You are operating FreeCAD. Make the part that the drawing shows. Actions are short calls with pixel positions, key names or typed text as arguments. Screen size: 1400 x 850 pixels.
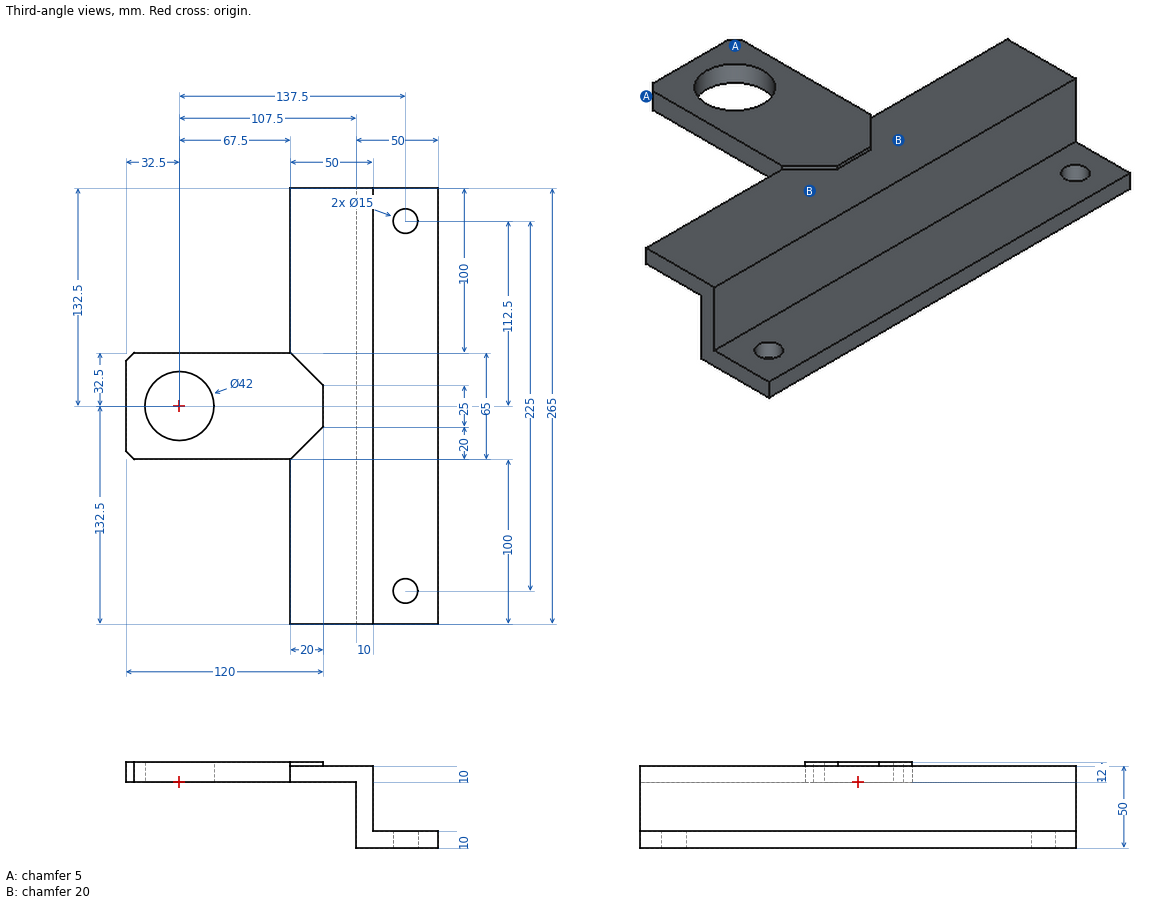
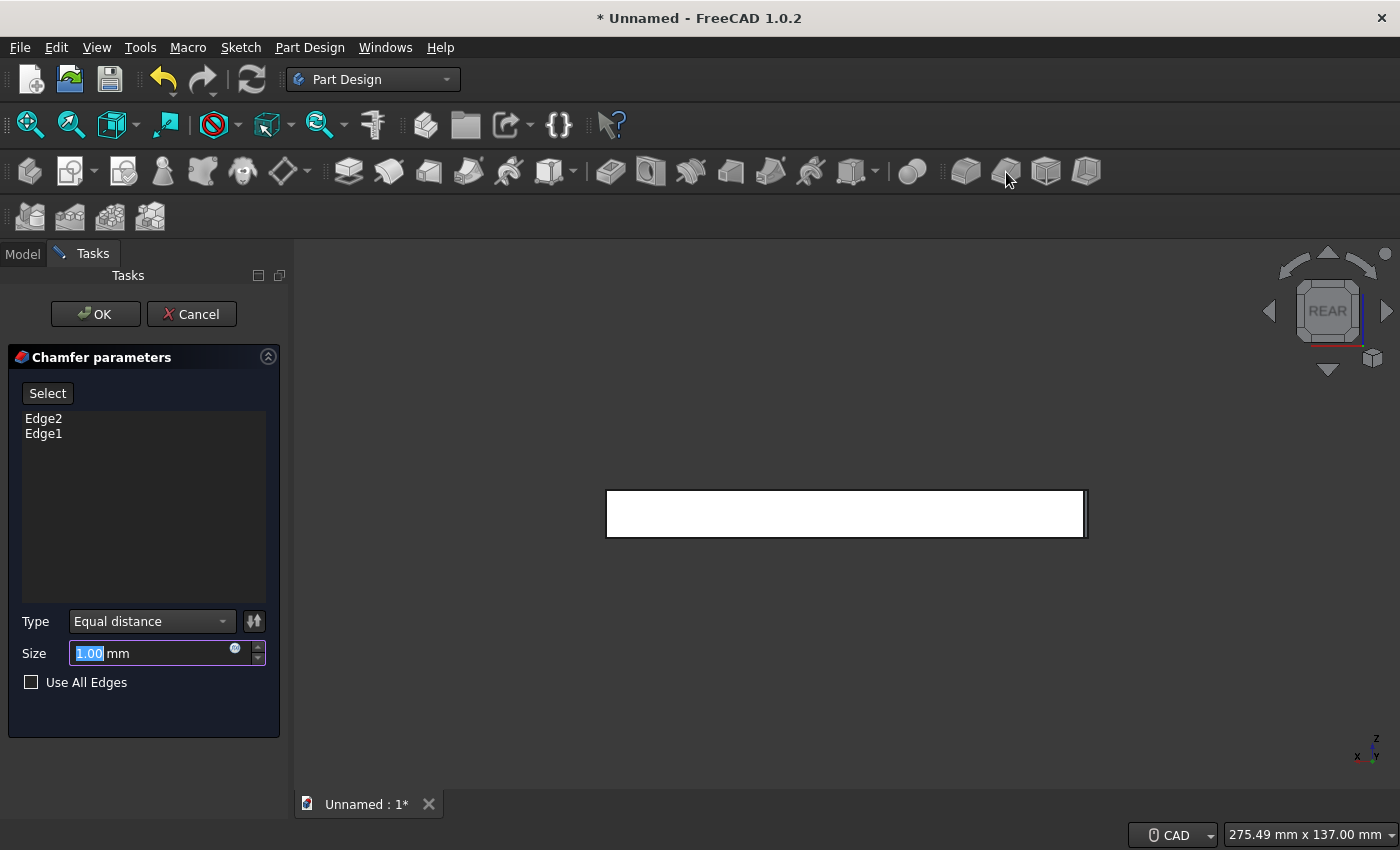
text(5)
key(Tab)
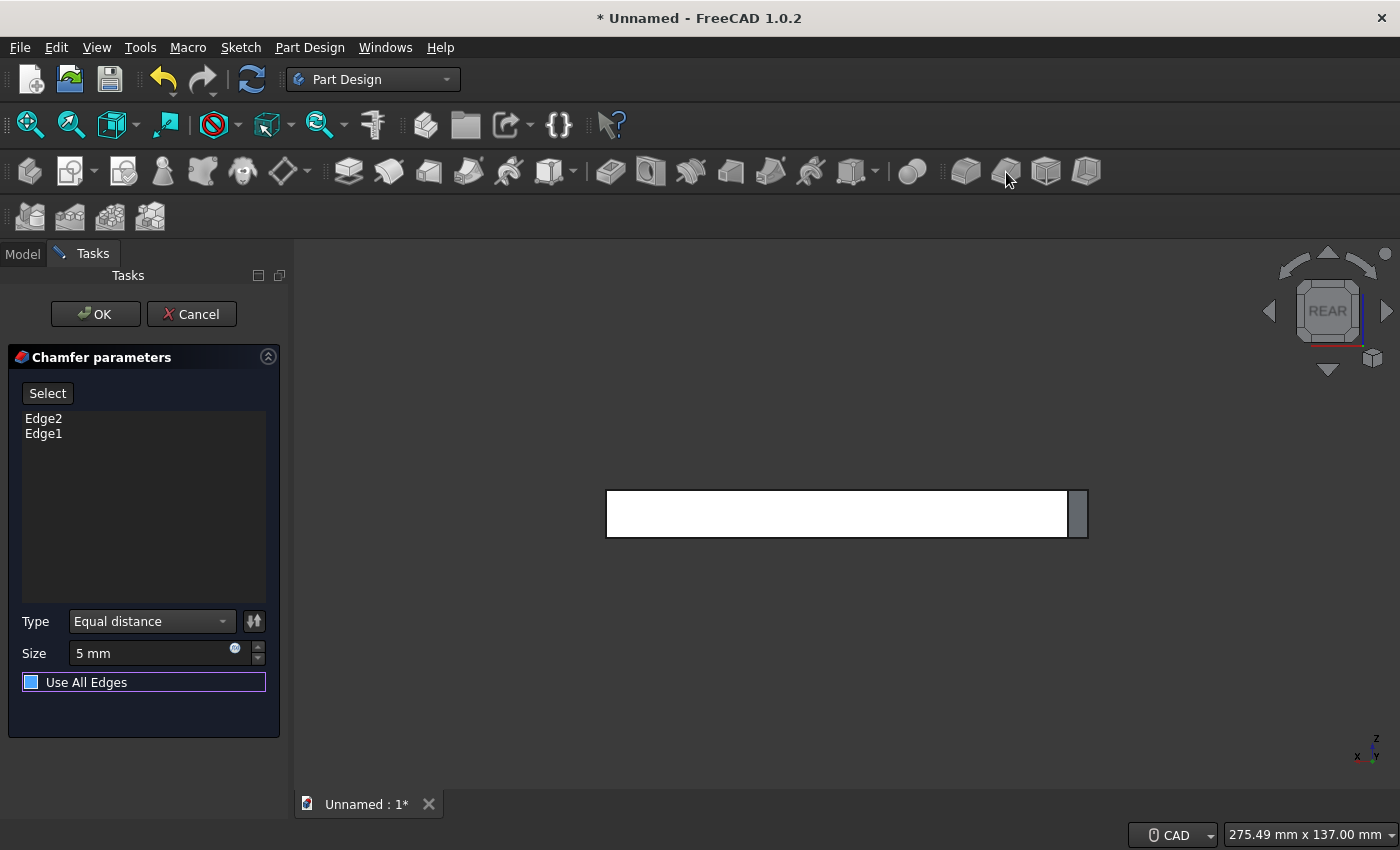
click(96, 314)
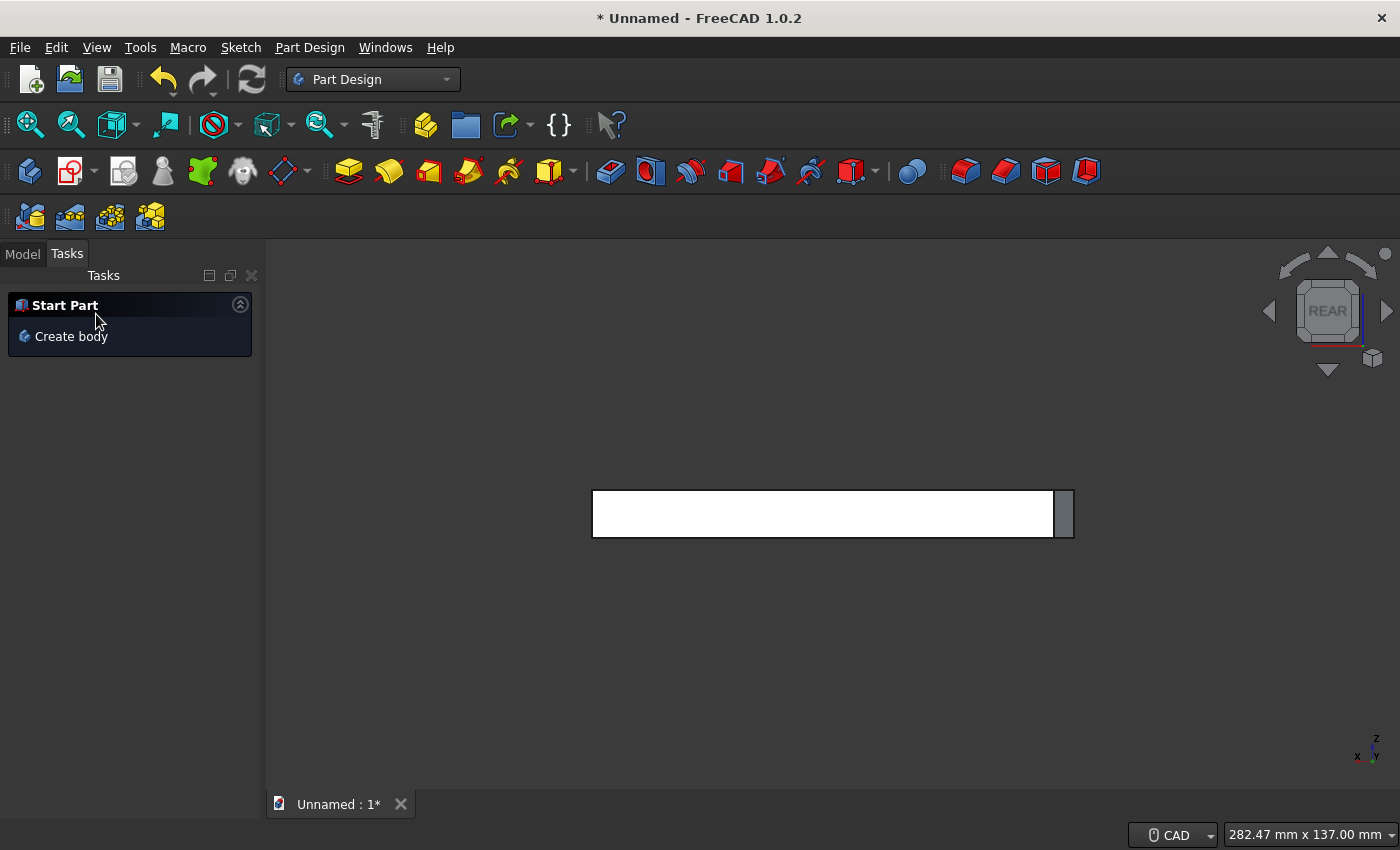
key(v)
key(f)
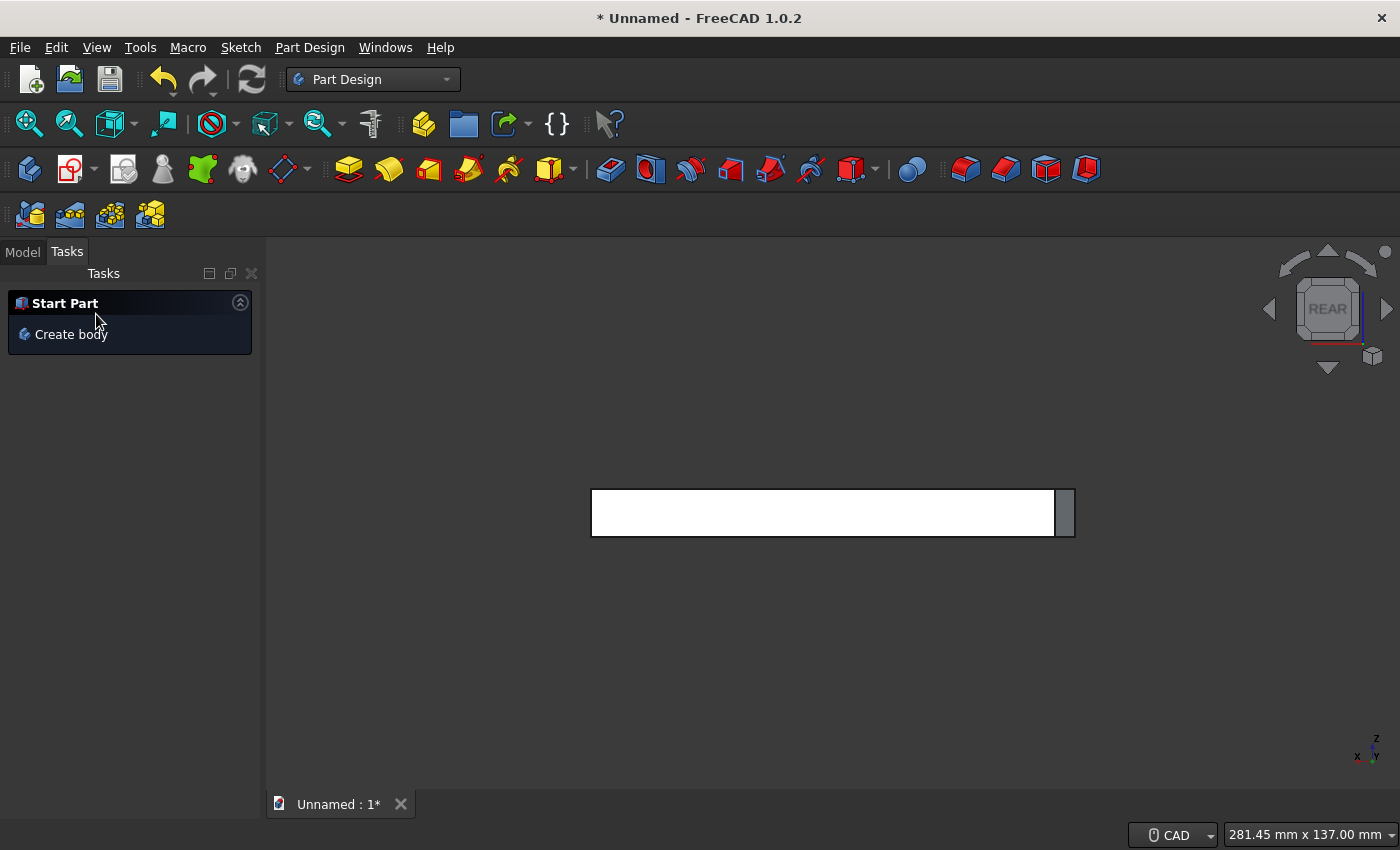
click(591, 512)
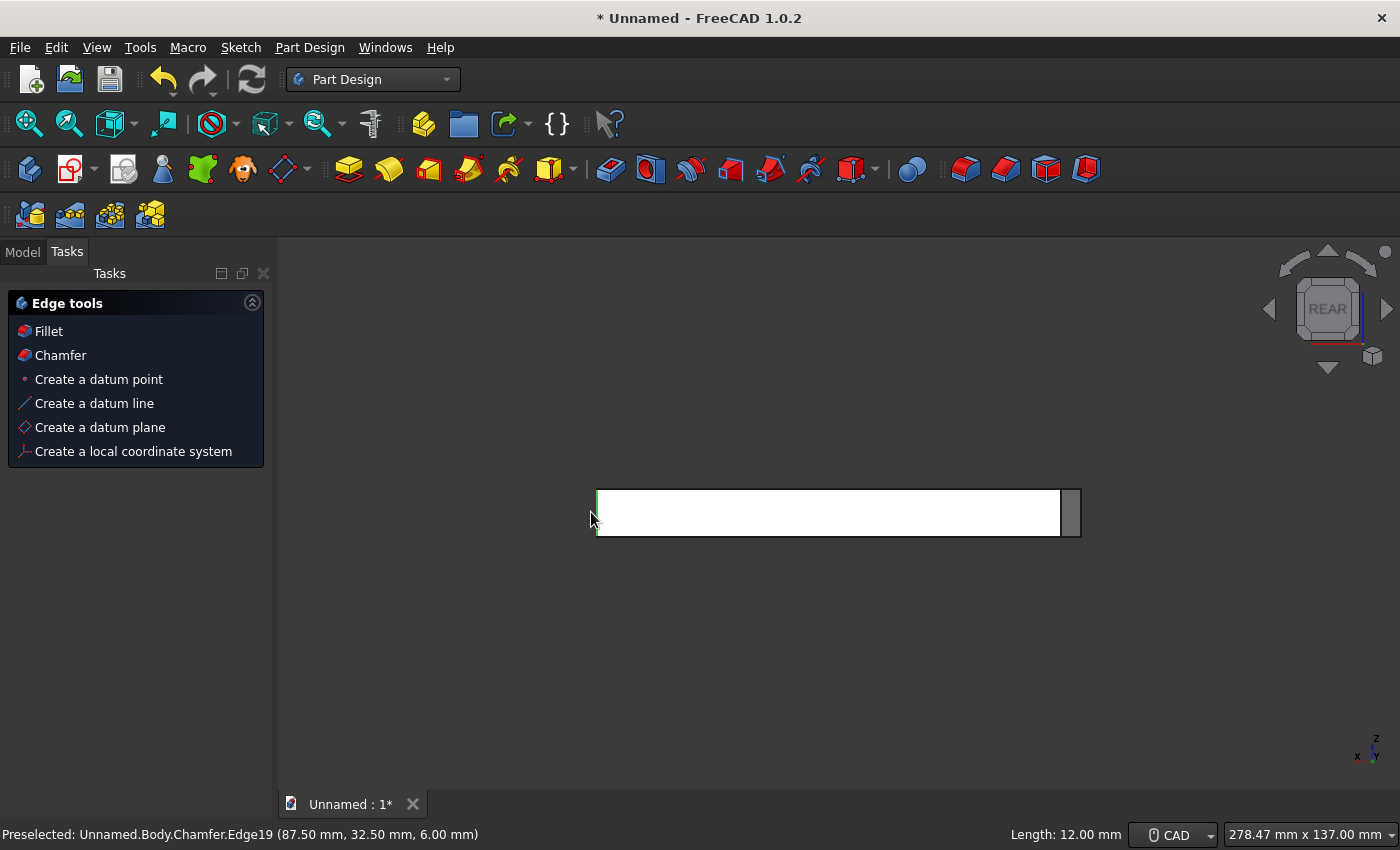
key(0)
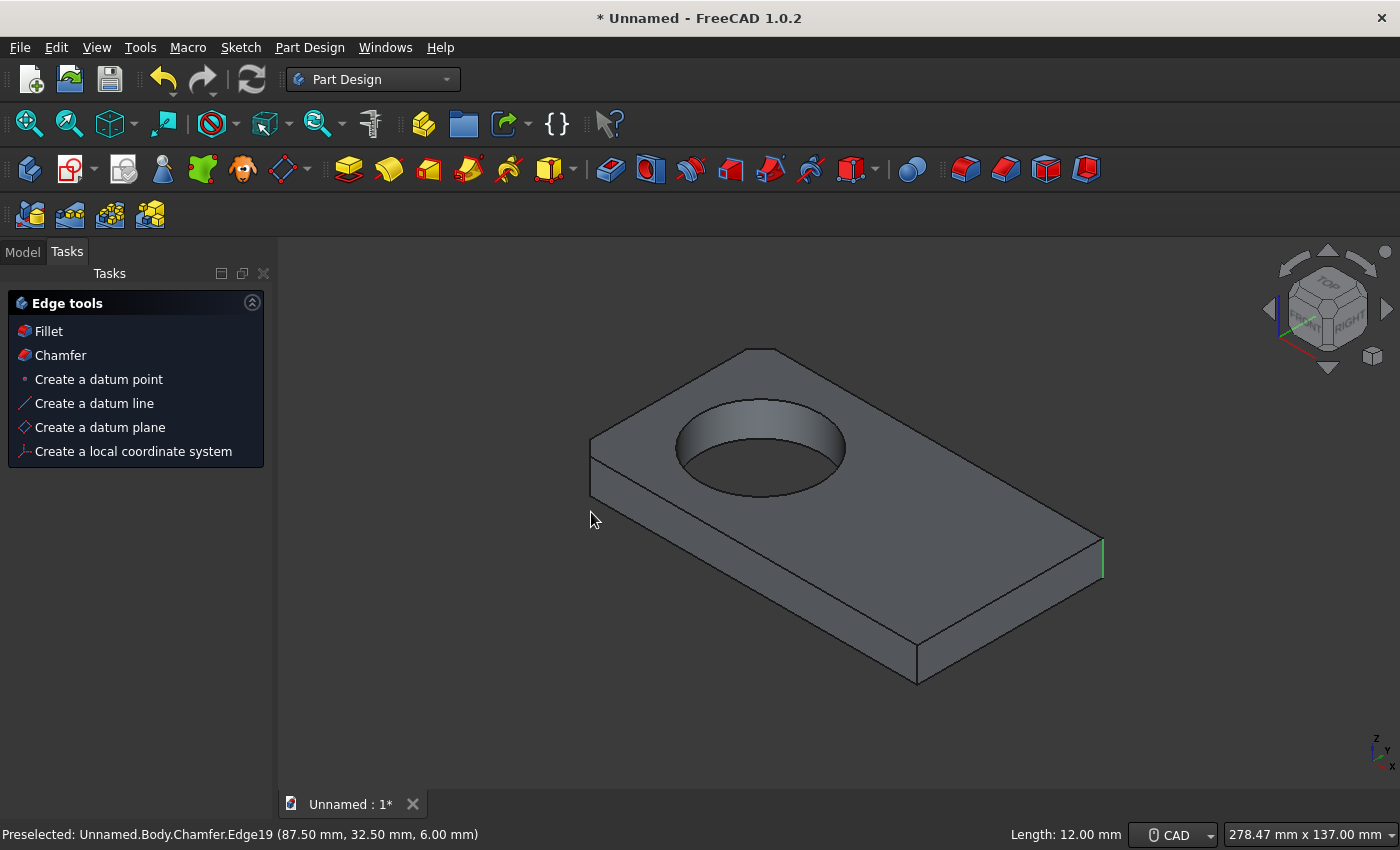
click(917, 664, ctrl)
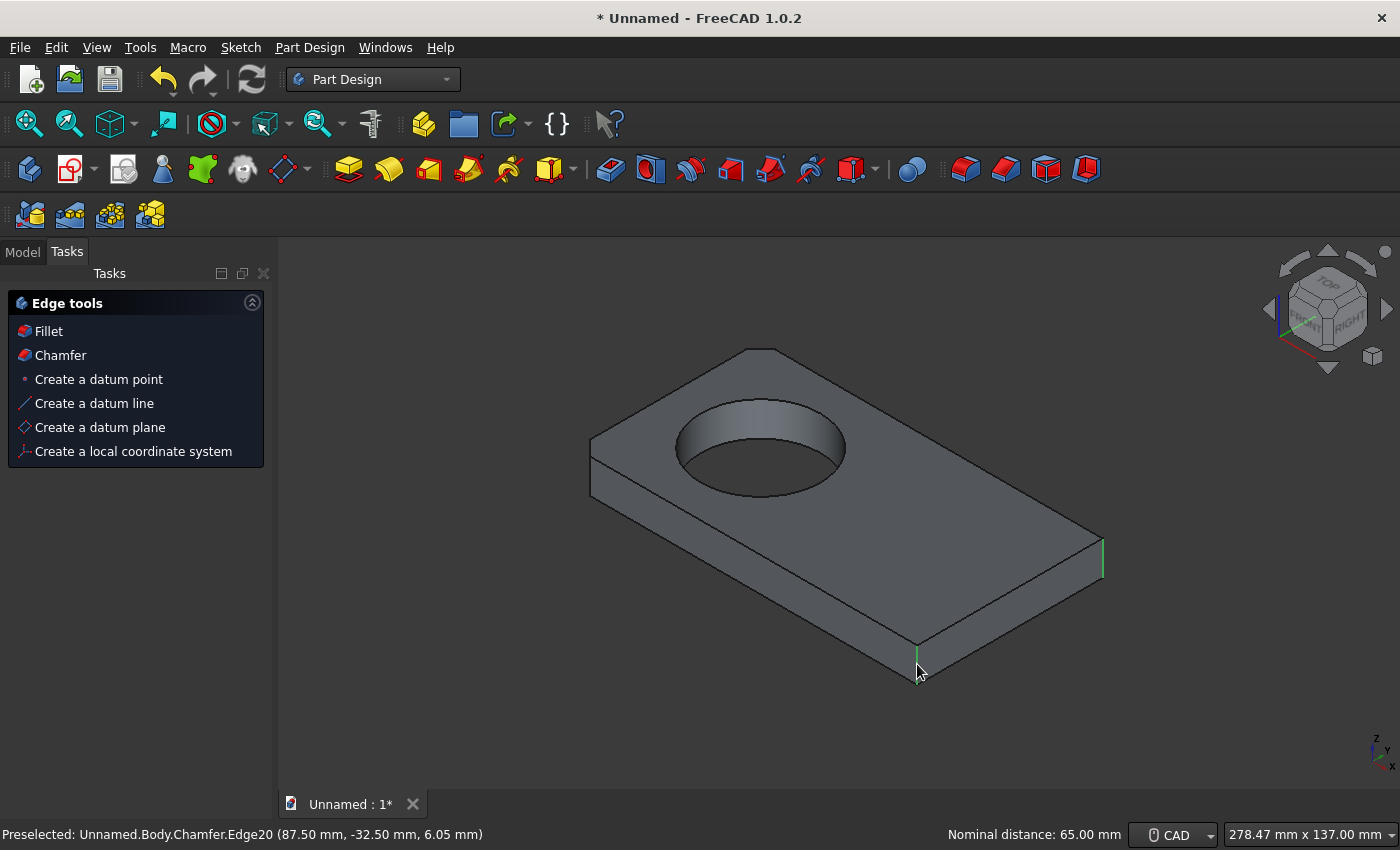
click(1006, 170)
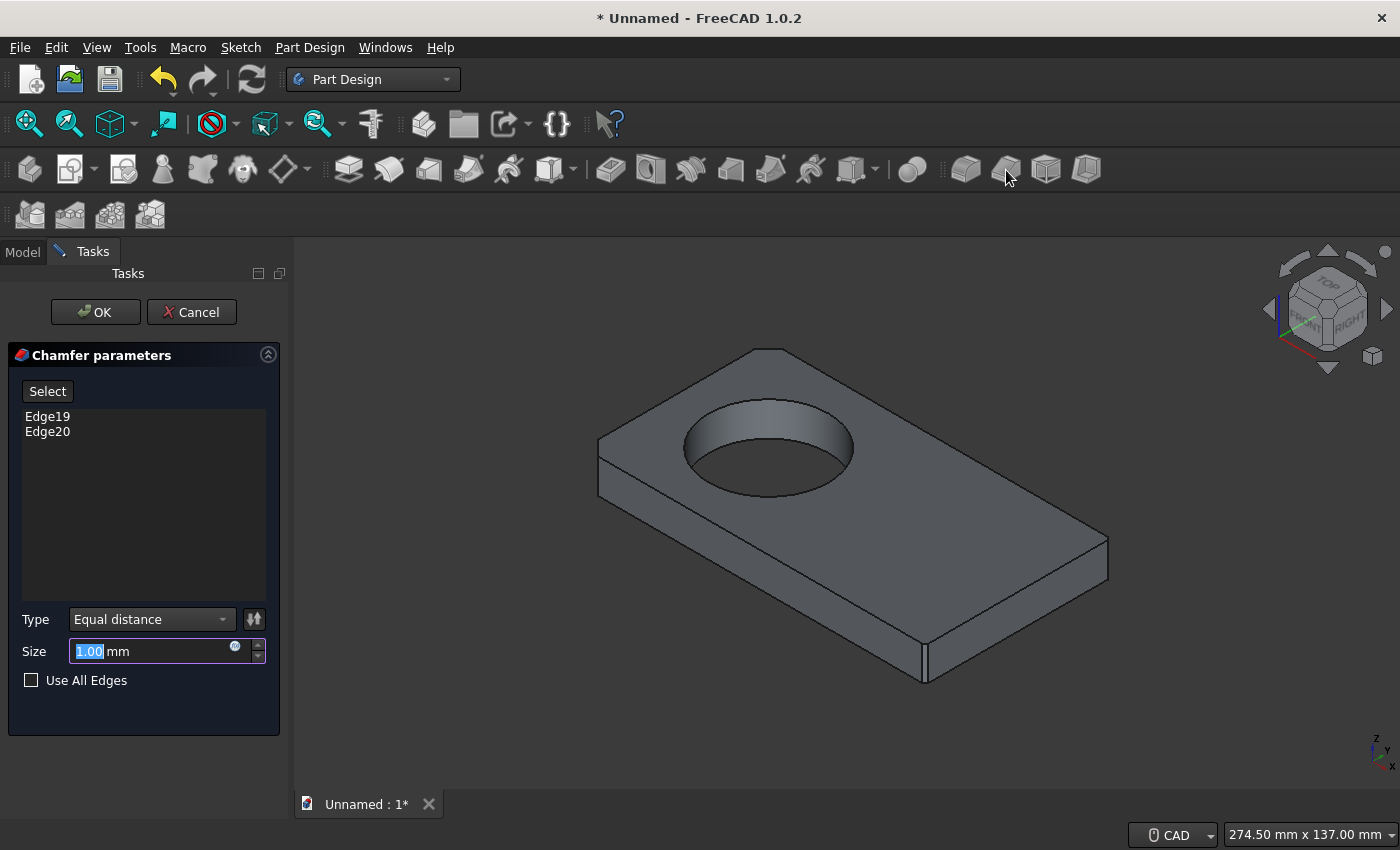
text(20)
key(Tab)